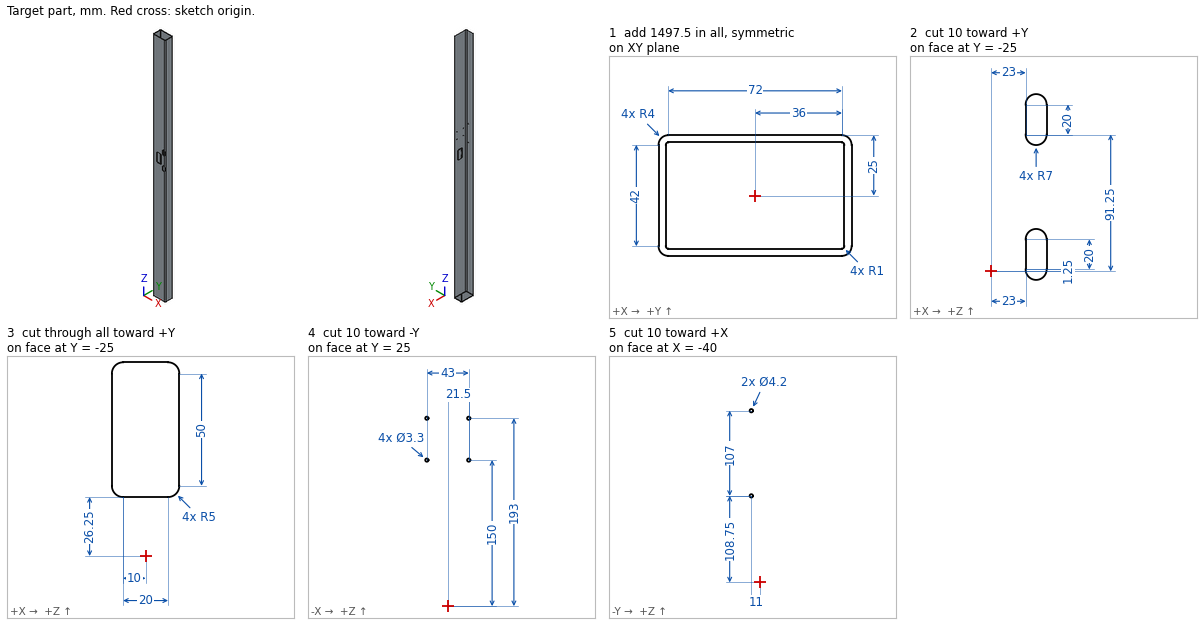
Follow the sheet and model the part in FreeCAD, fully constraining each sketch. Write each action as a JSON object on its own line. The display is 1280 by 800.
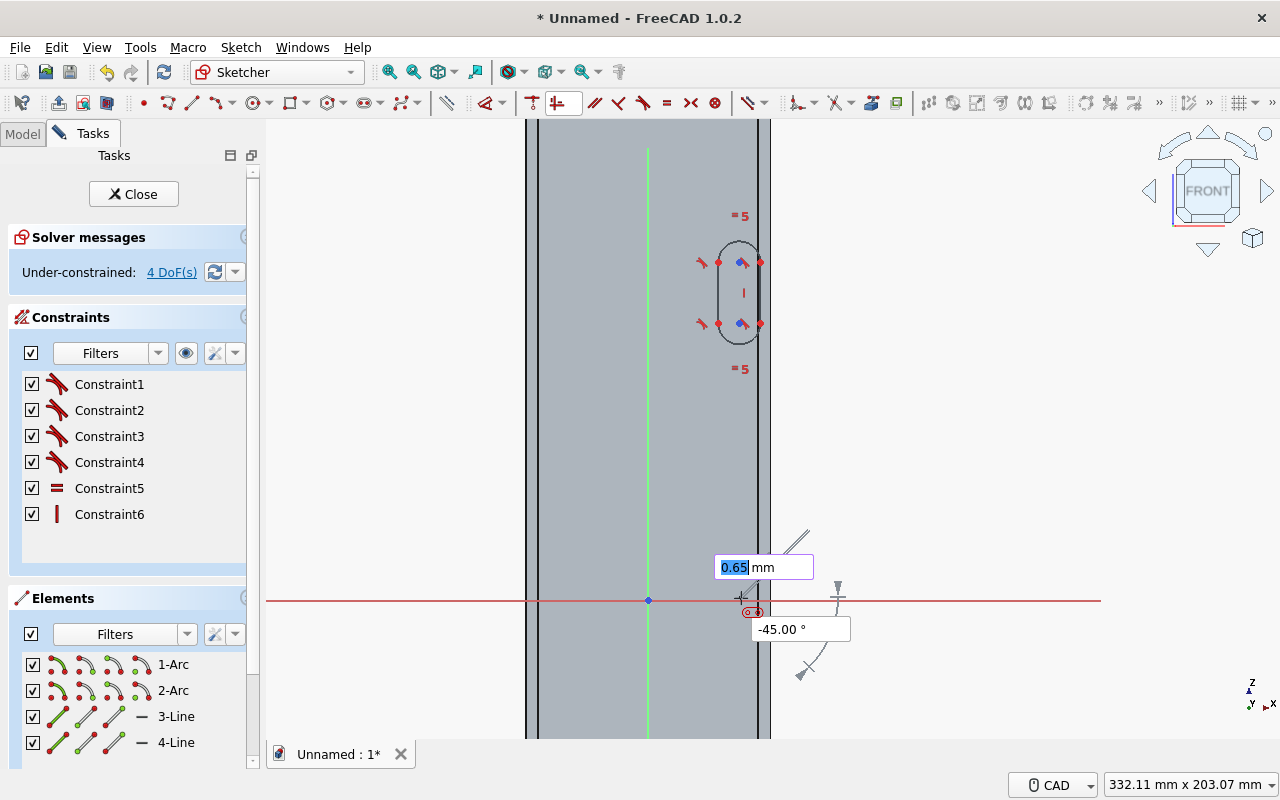
{"action": "left_click", "coordinate": [740, 536]}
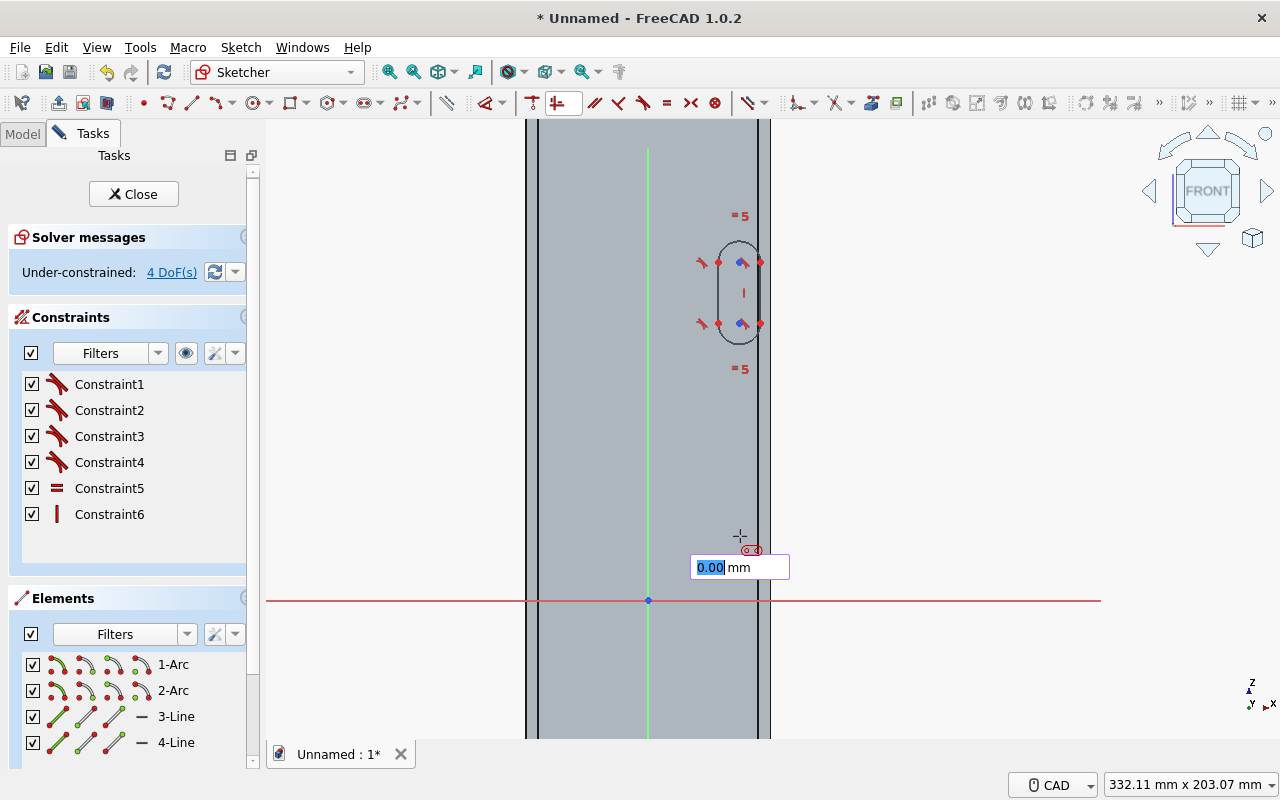
{"action": "left_click", "coordinate": [719, 567]}
{"action": "key", "text": "Escape"}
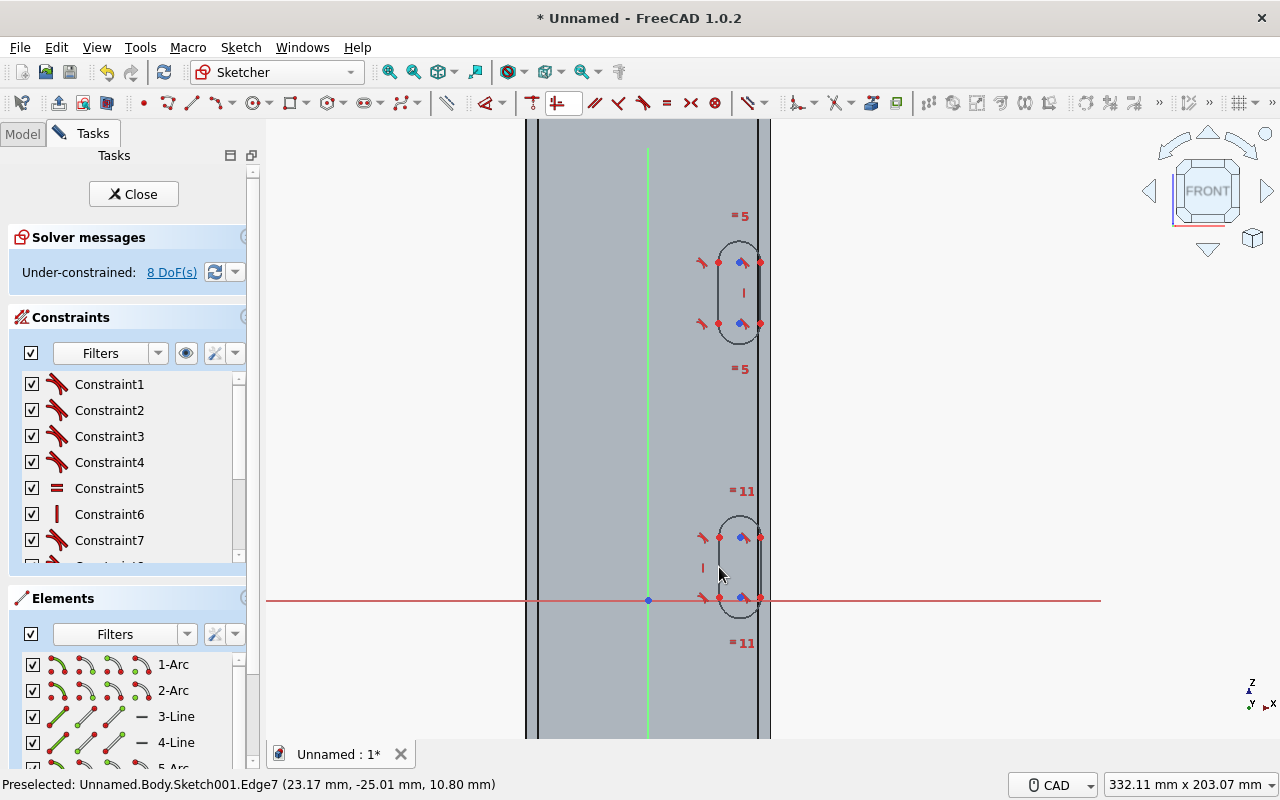
{"action": "left_click", "coordinate": [727, 340]}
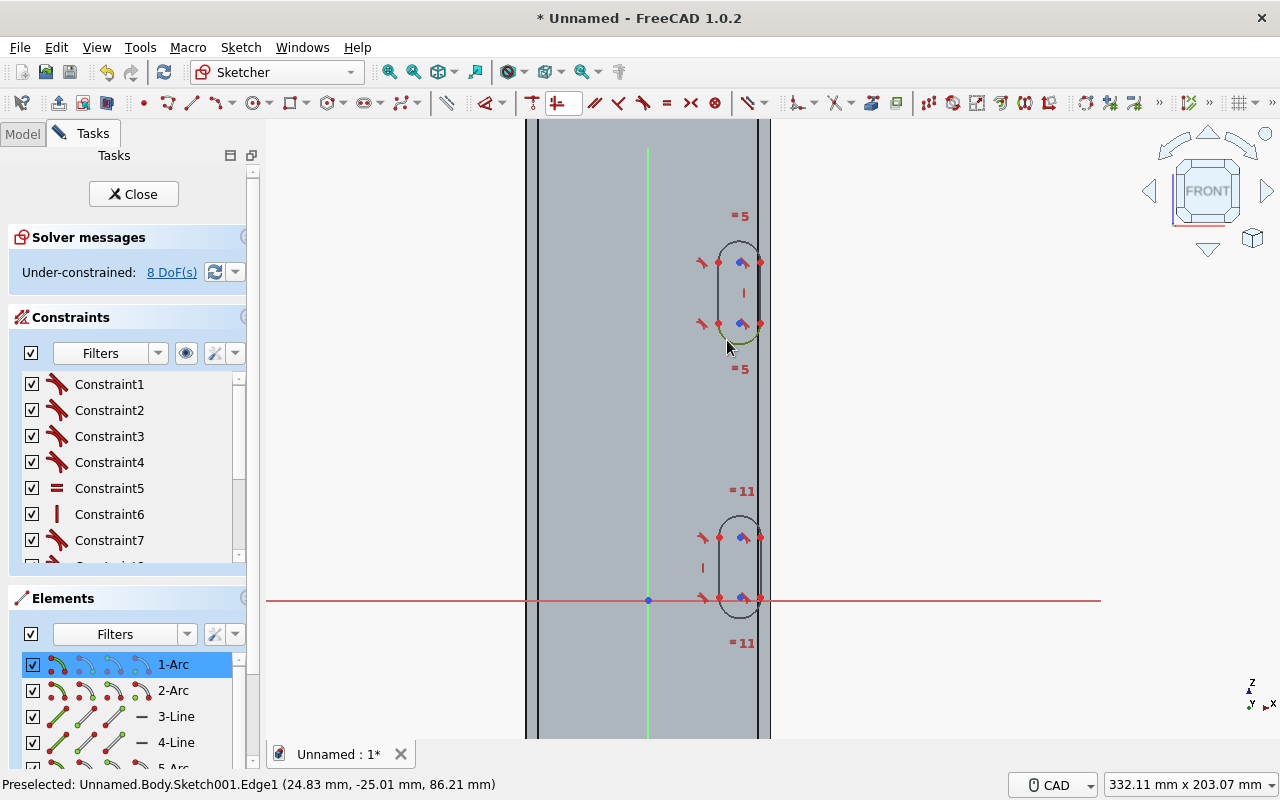
{"action": "left_click", "coordinate": [728, 614]}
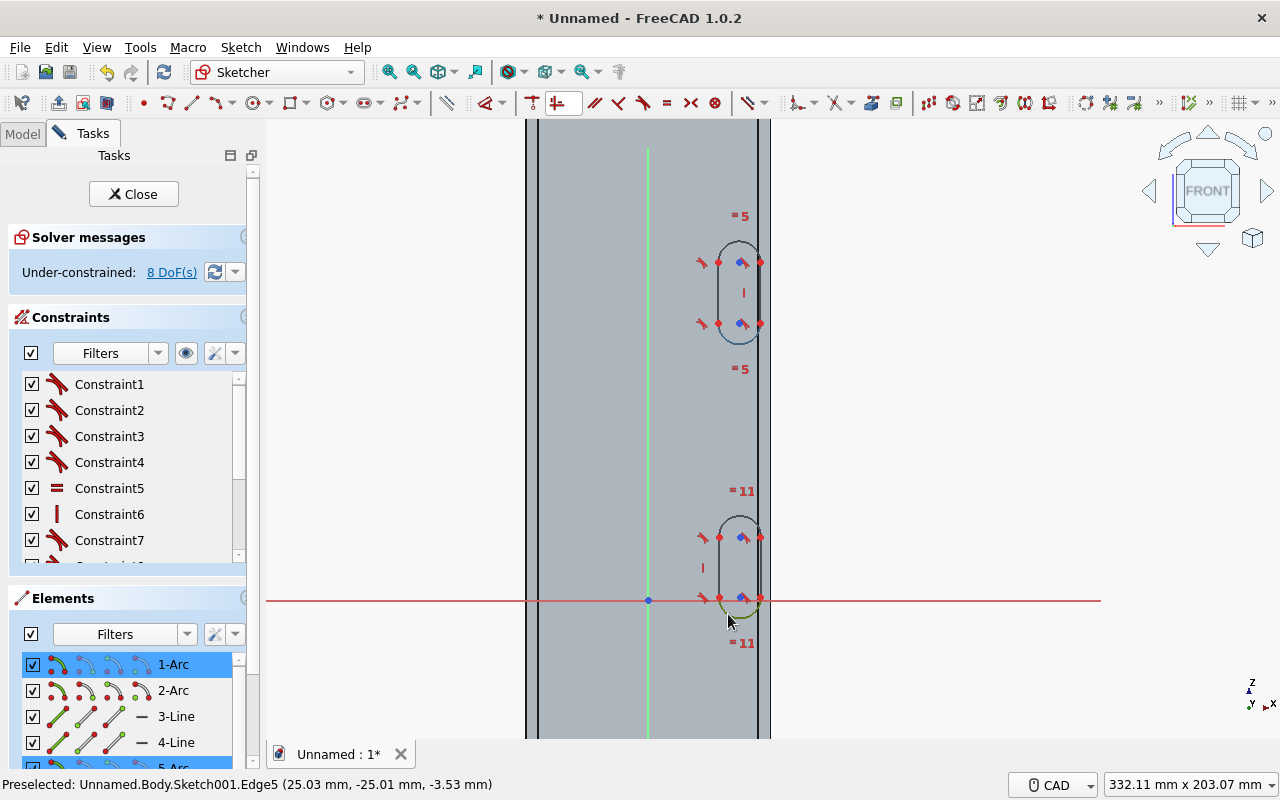
{"action": "left_click", "coordinate": [668, 104]}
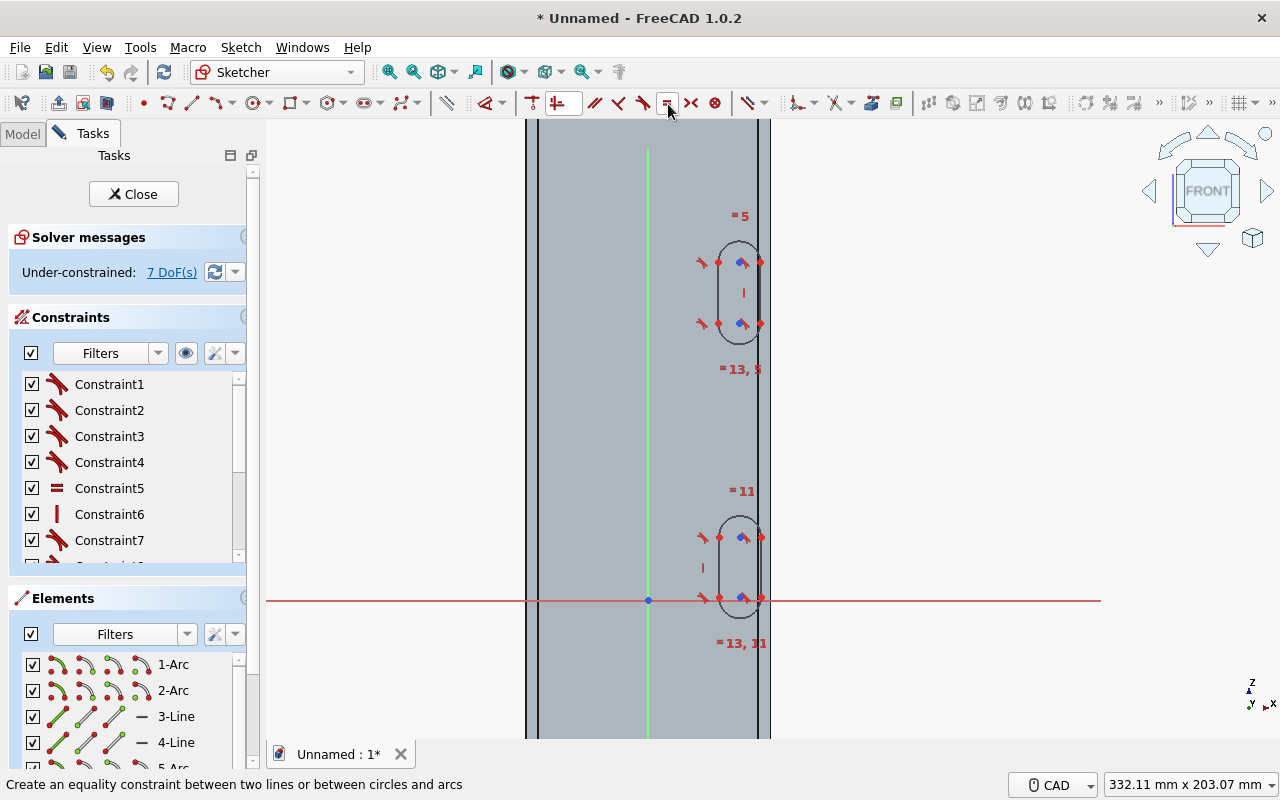
{"action": "key", "text": "d"}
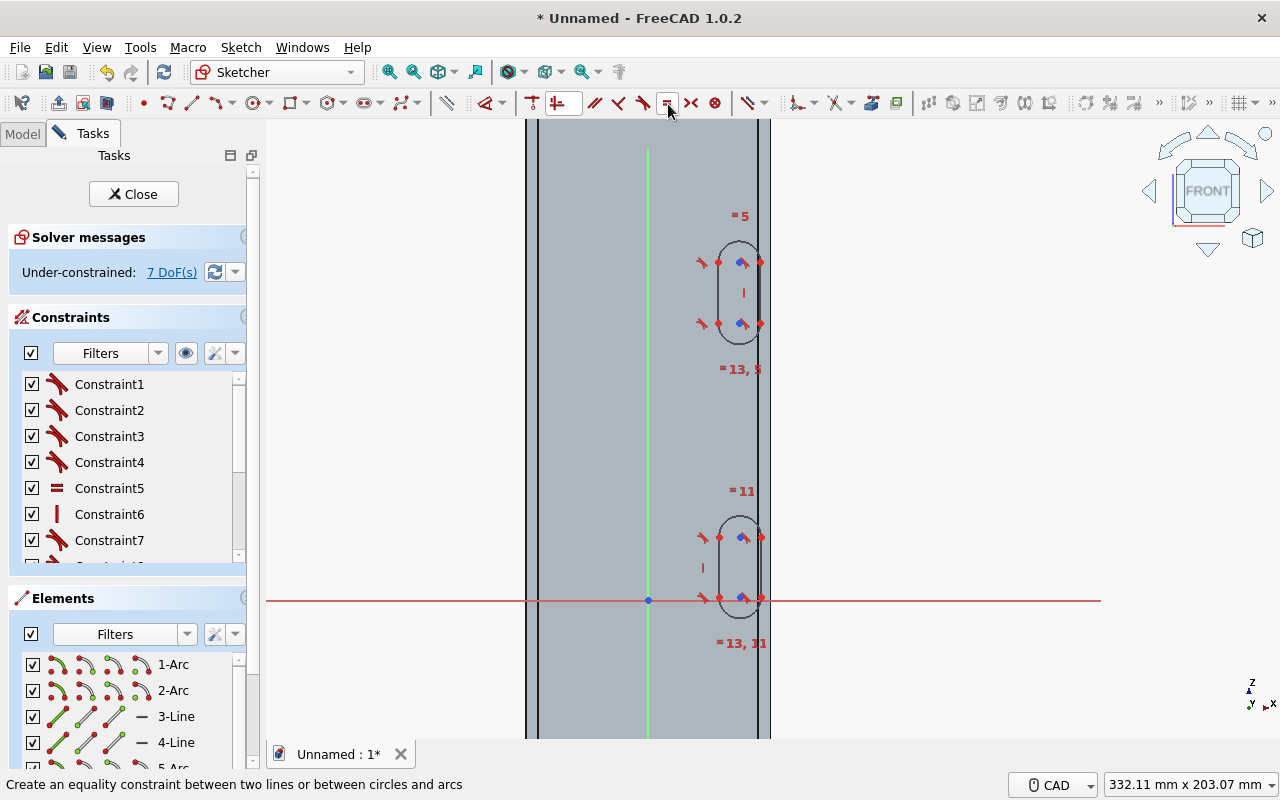
{"action": "scroll", "coordinate": [727, 340], "scroll_direction": "up", "scroll_amount": 4}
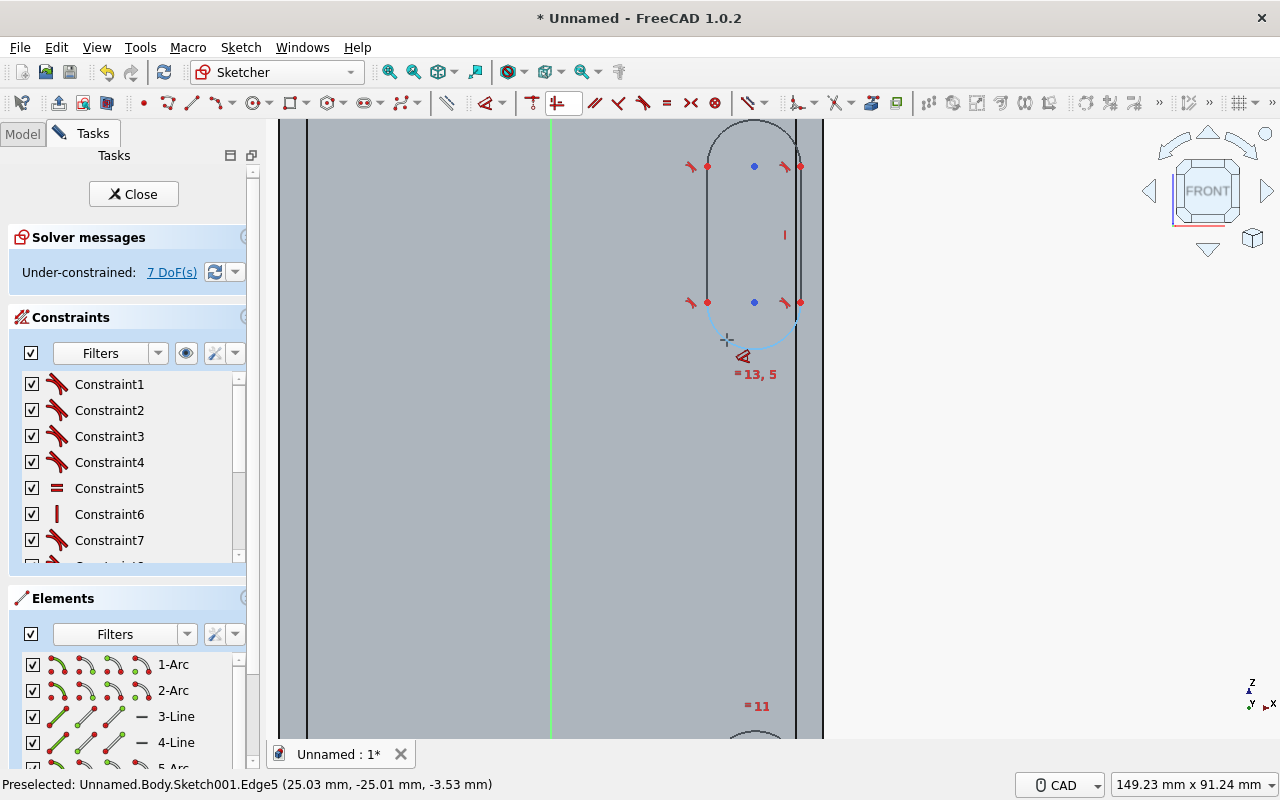
{"action": "left_click", "coordinate": [727, 340]}
{"action": "left_click", "coordinate": [708, 366]}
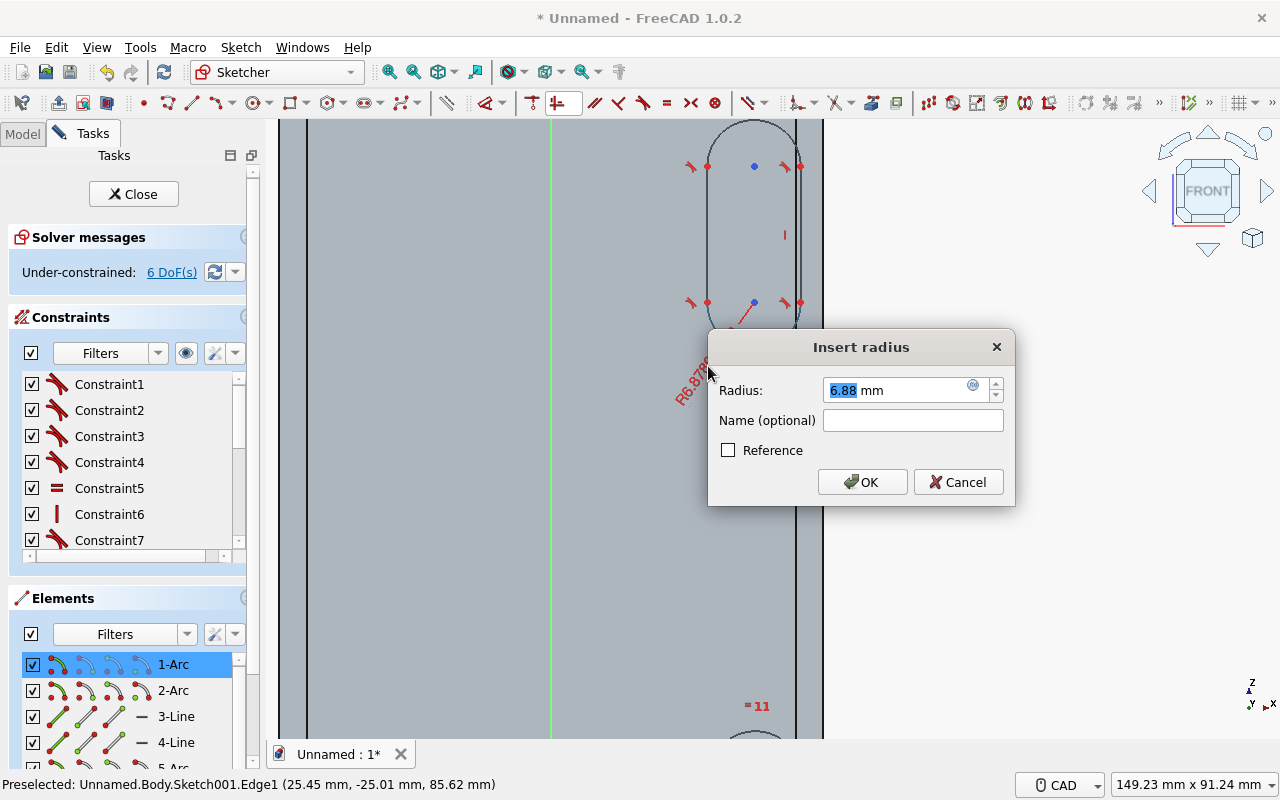
{"action": "type", "text": "7"}
{"action": "key", "text": "Return"}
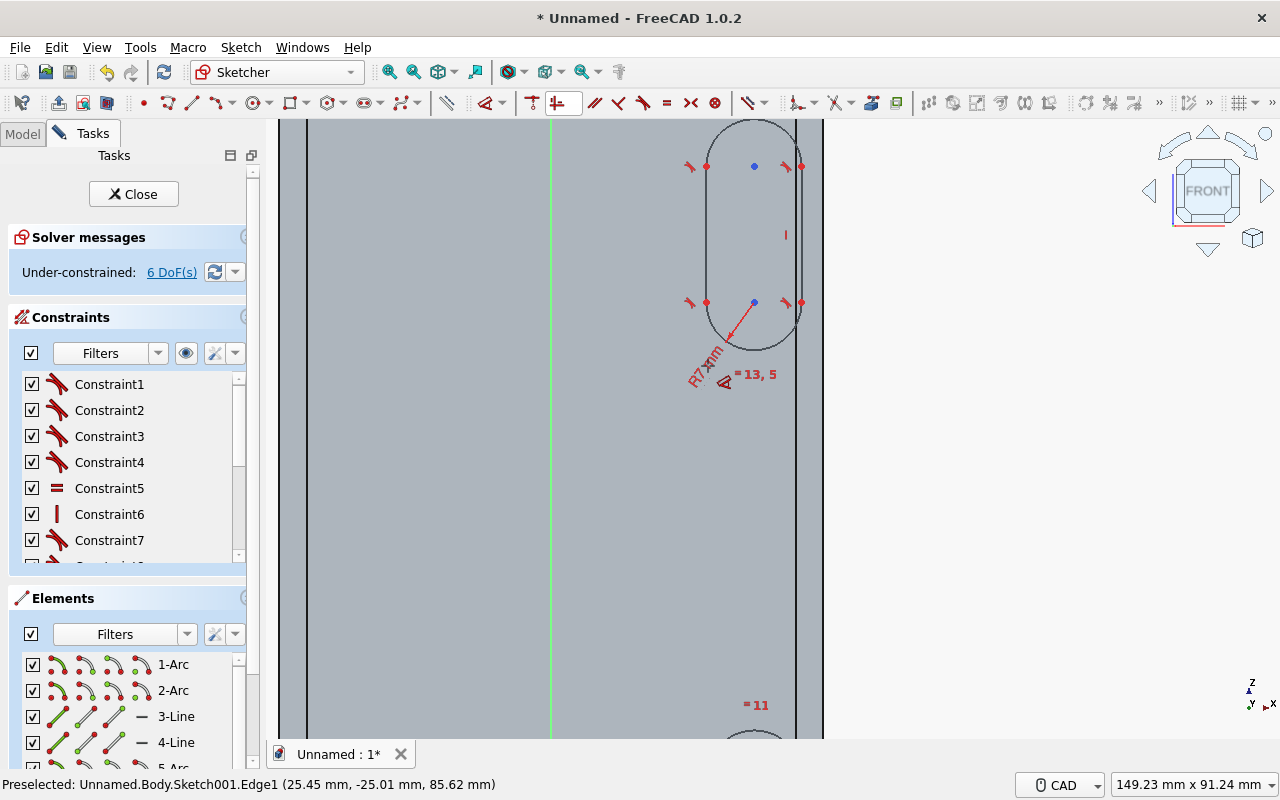
{"action": "left_click", "coordinate": [706, 262]}
{"action": "left_click", "coordinate": [740, 235]}